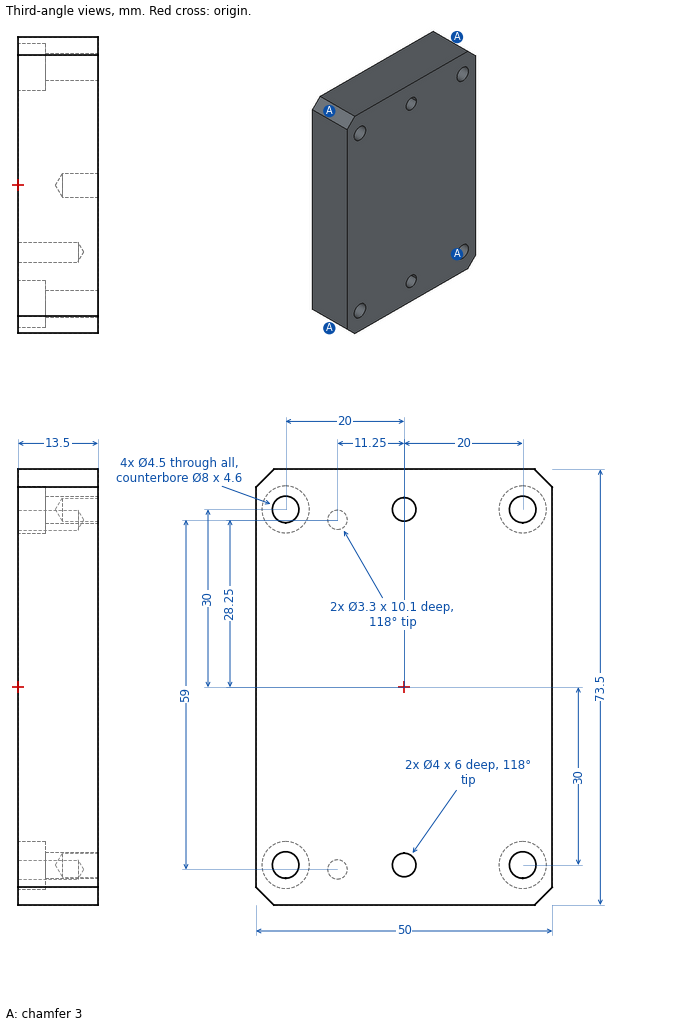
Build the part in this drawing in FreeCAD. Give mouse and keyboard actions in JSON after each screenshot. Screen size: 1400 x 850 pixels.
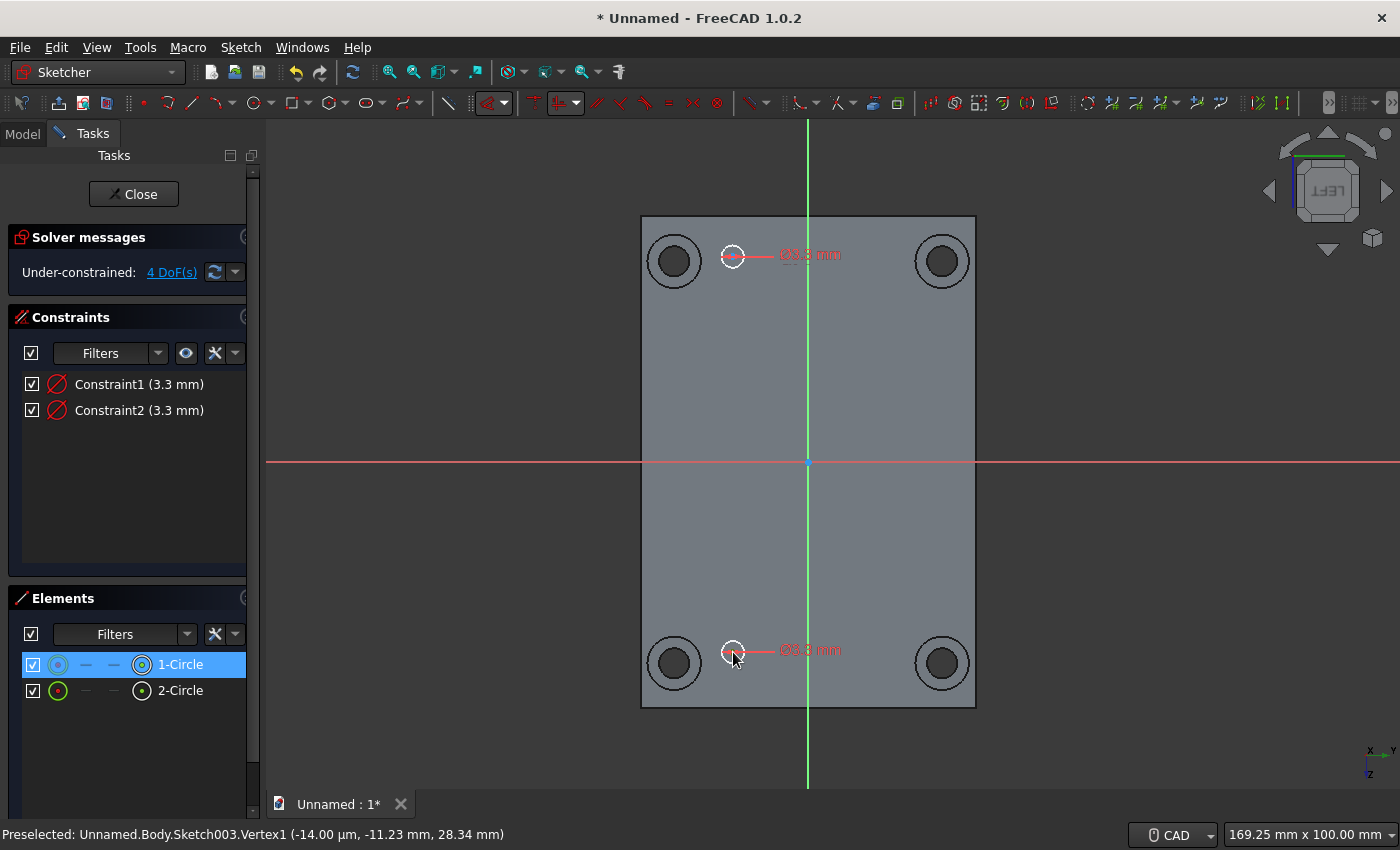
{"action": "left_click", "coordinate": [733, 257]}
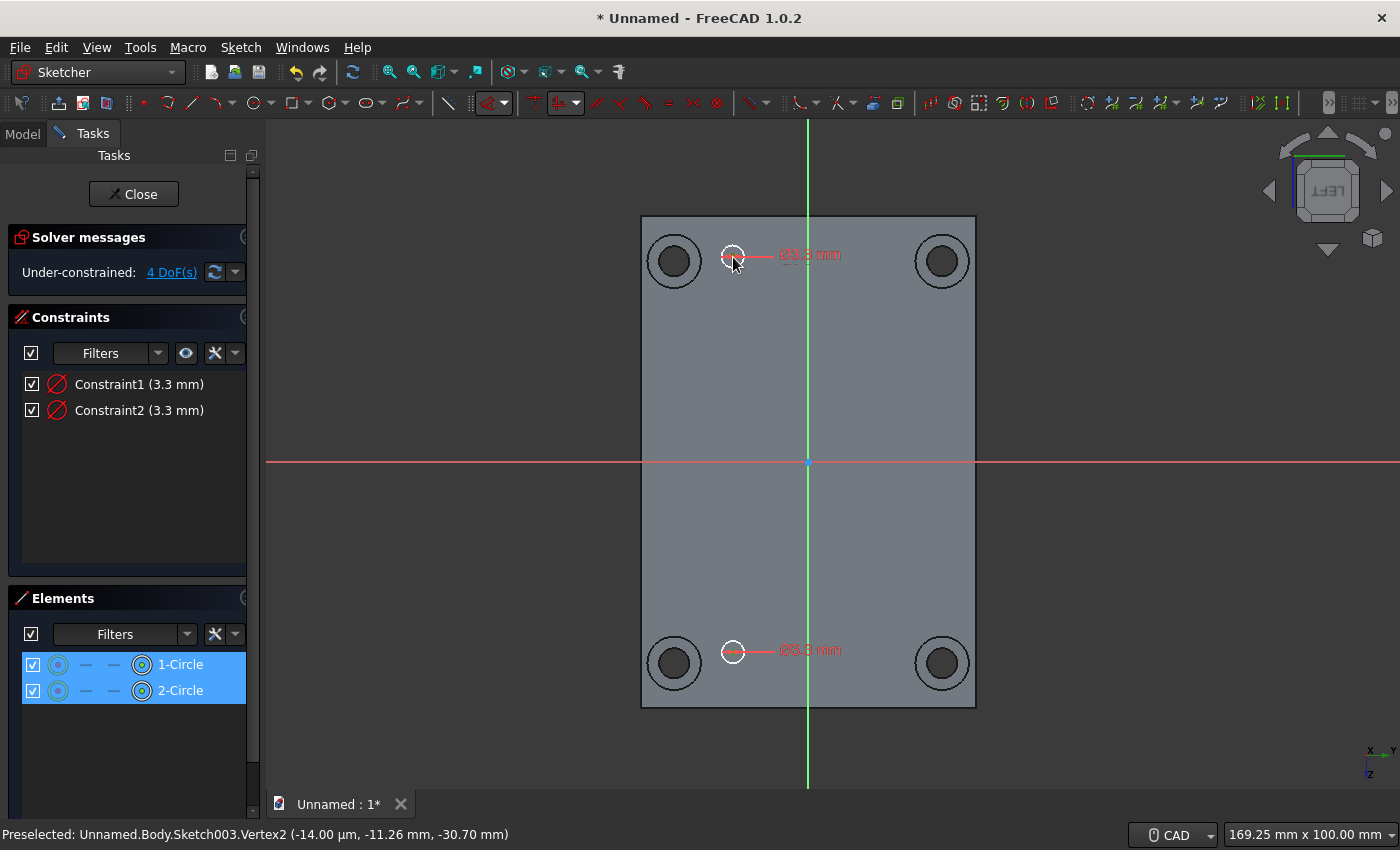
{"action": "key", "text": "v"}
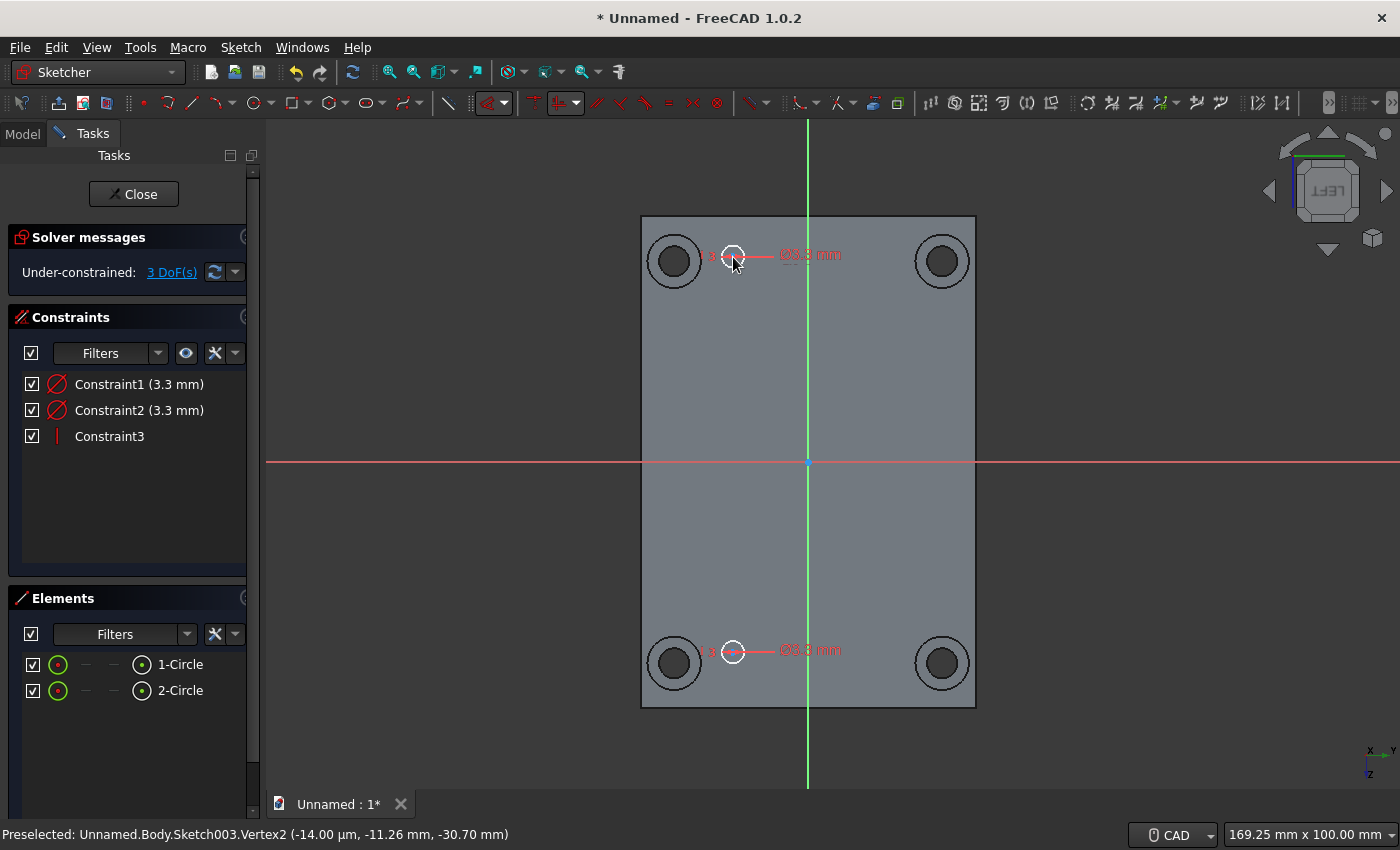
{"action": "left_click", "coordinate": [733, 652]}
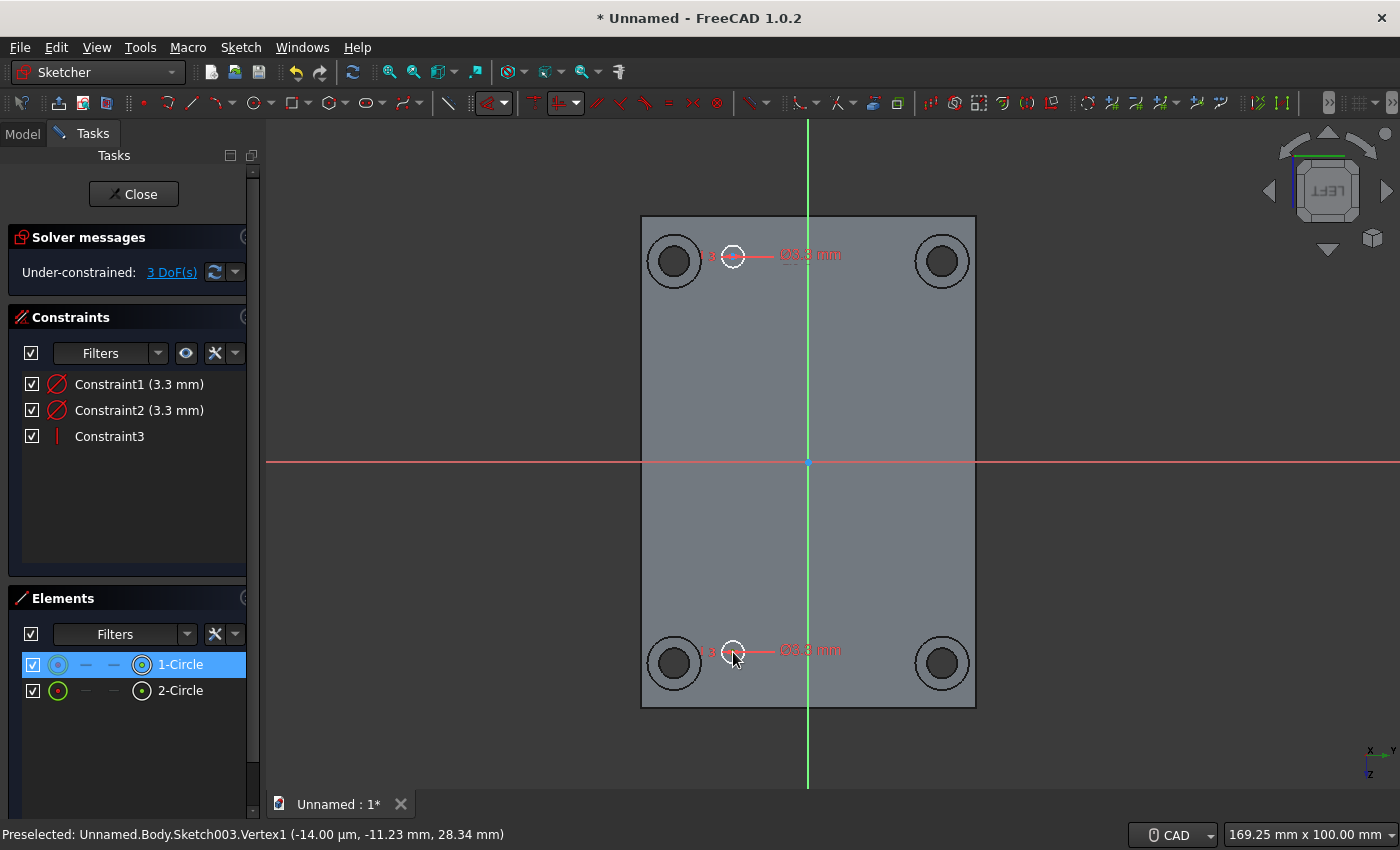
{"action": "left_click", "coordinate": [733, 257]}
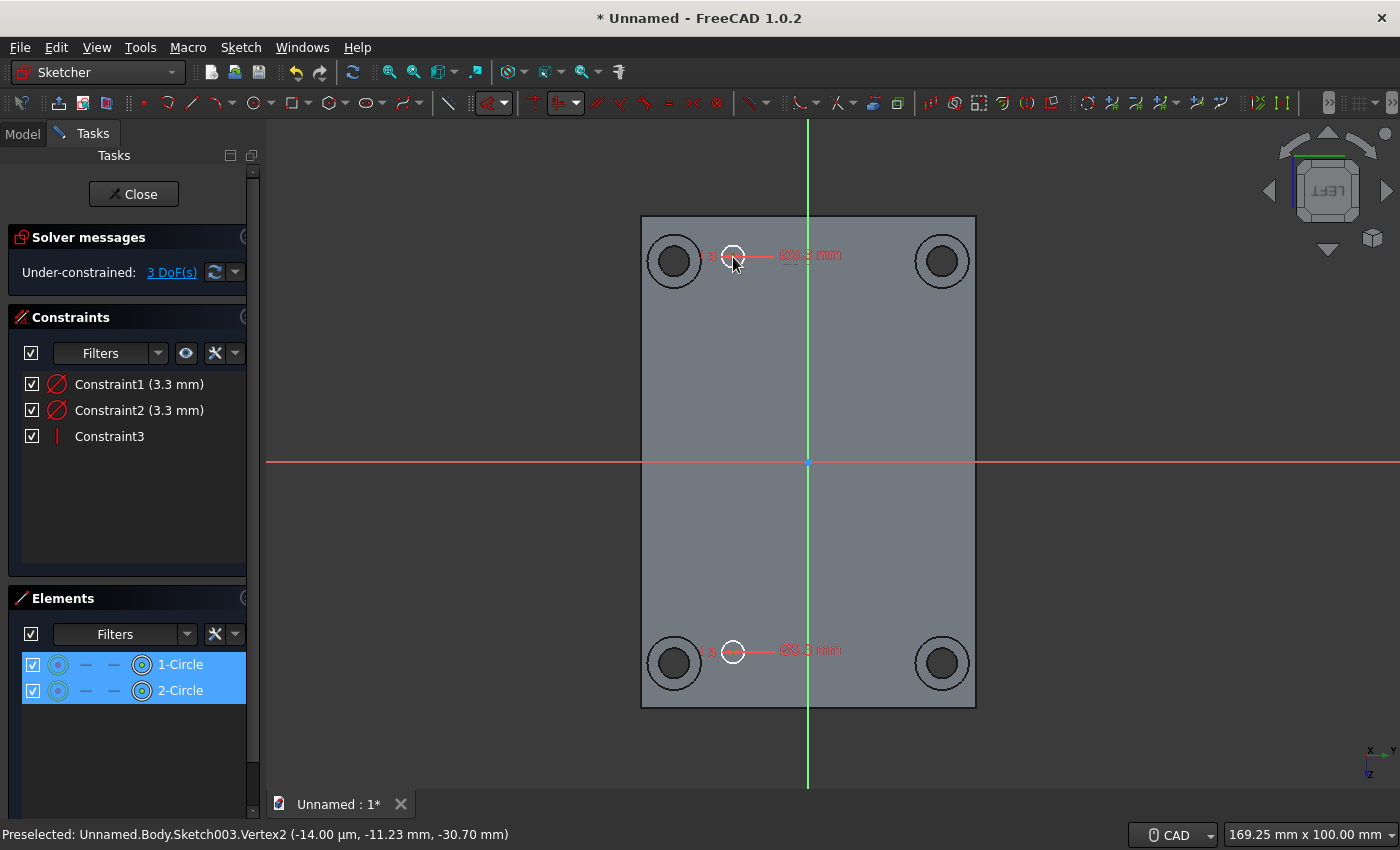
{"action": "left_click", "coordinate": [506, 104]}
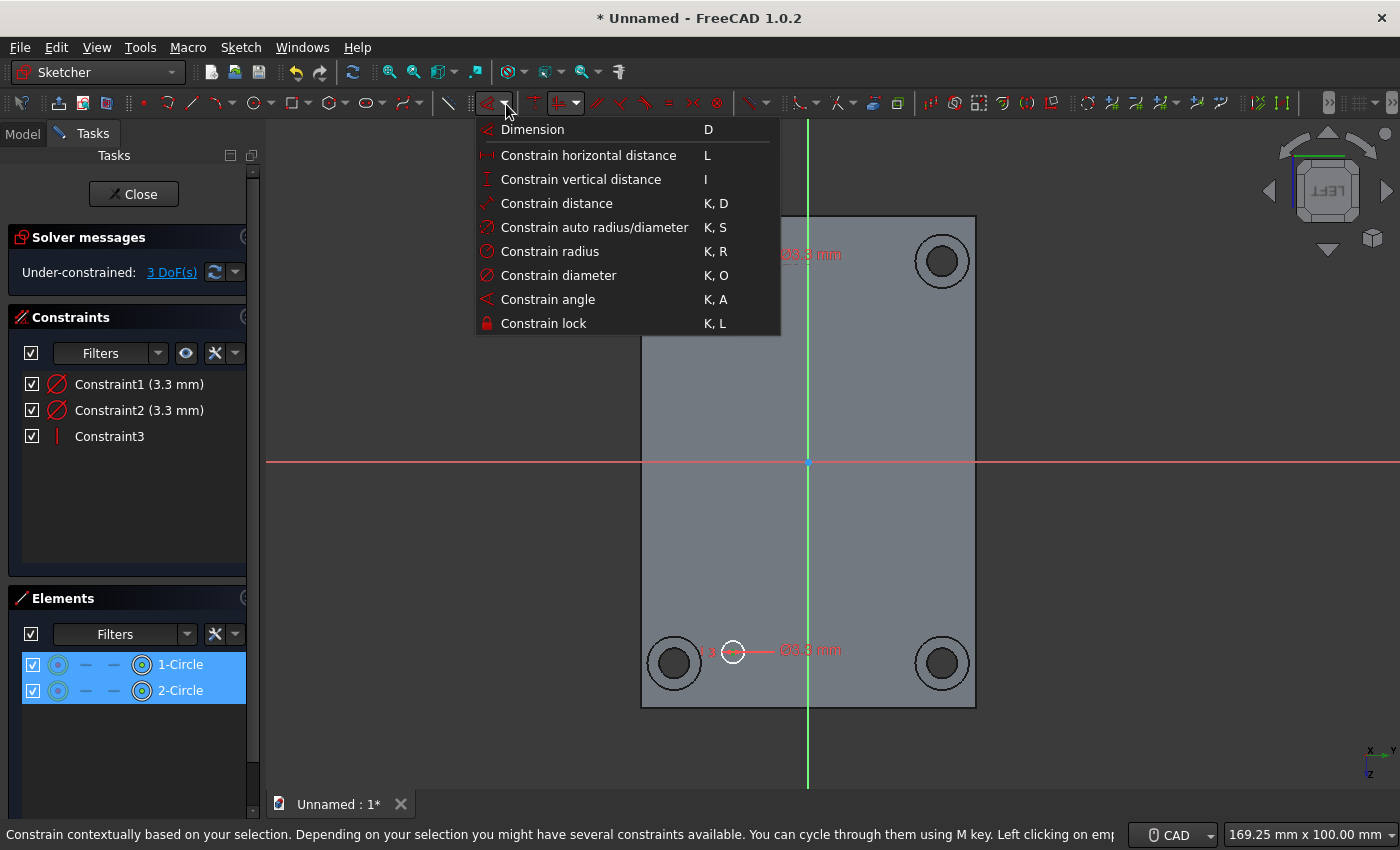
{"action": "left_click", "coordinate": [628, 179]}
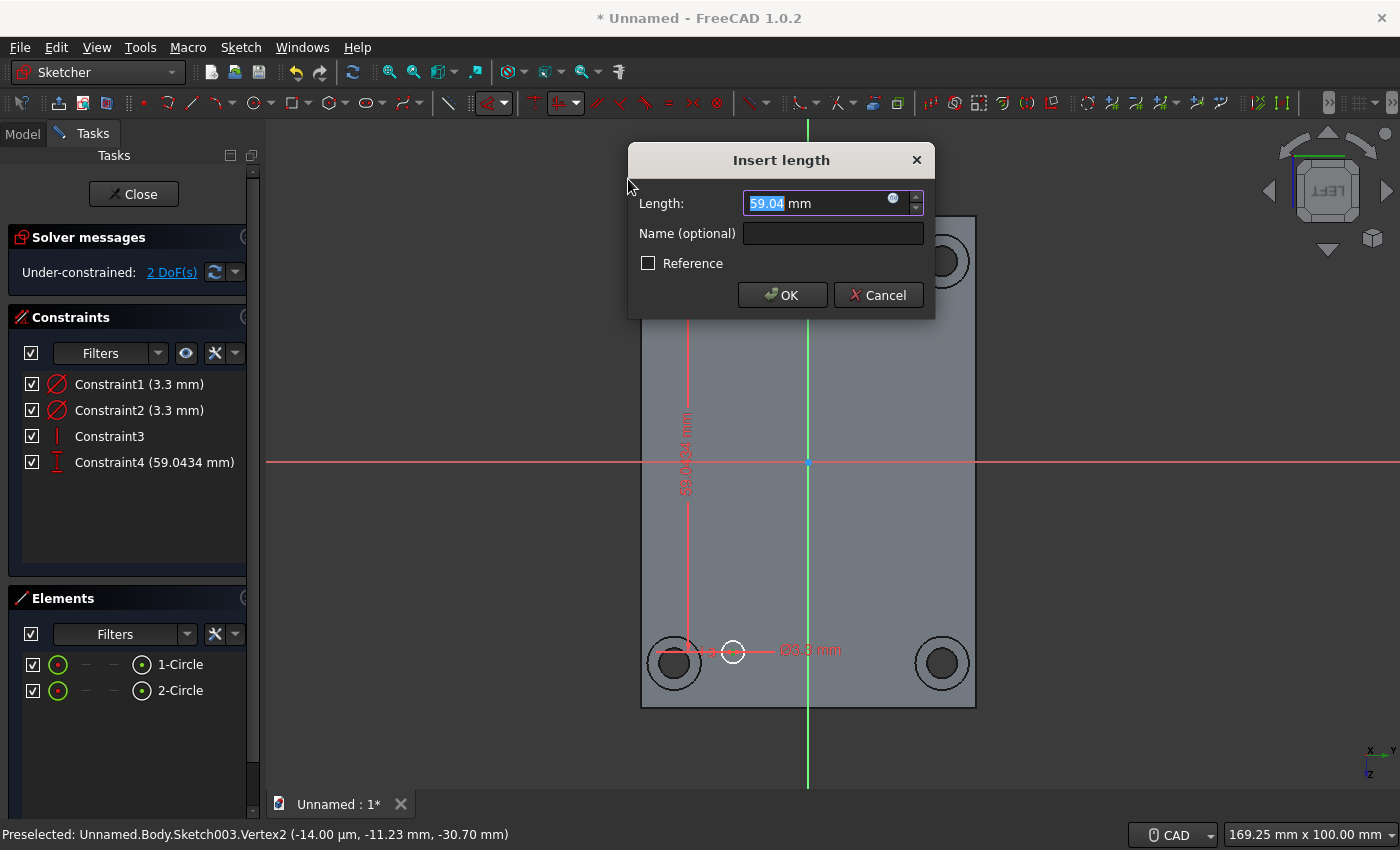
{"action": "type", "text": "59"}
{"action": "key", "text": "Return"}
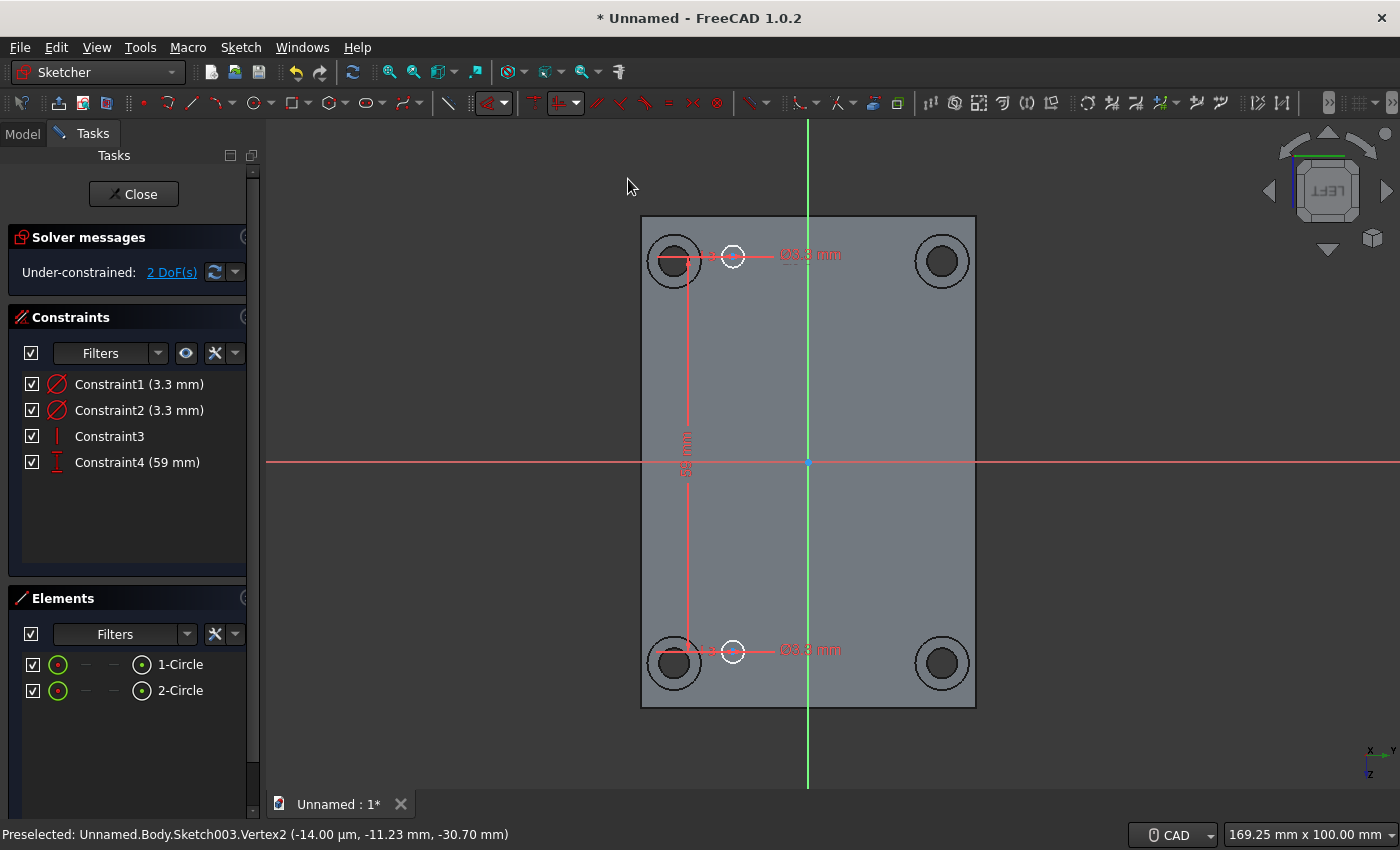
{"action": "left_click", "coordinate": [733, 652]}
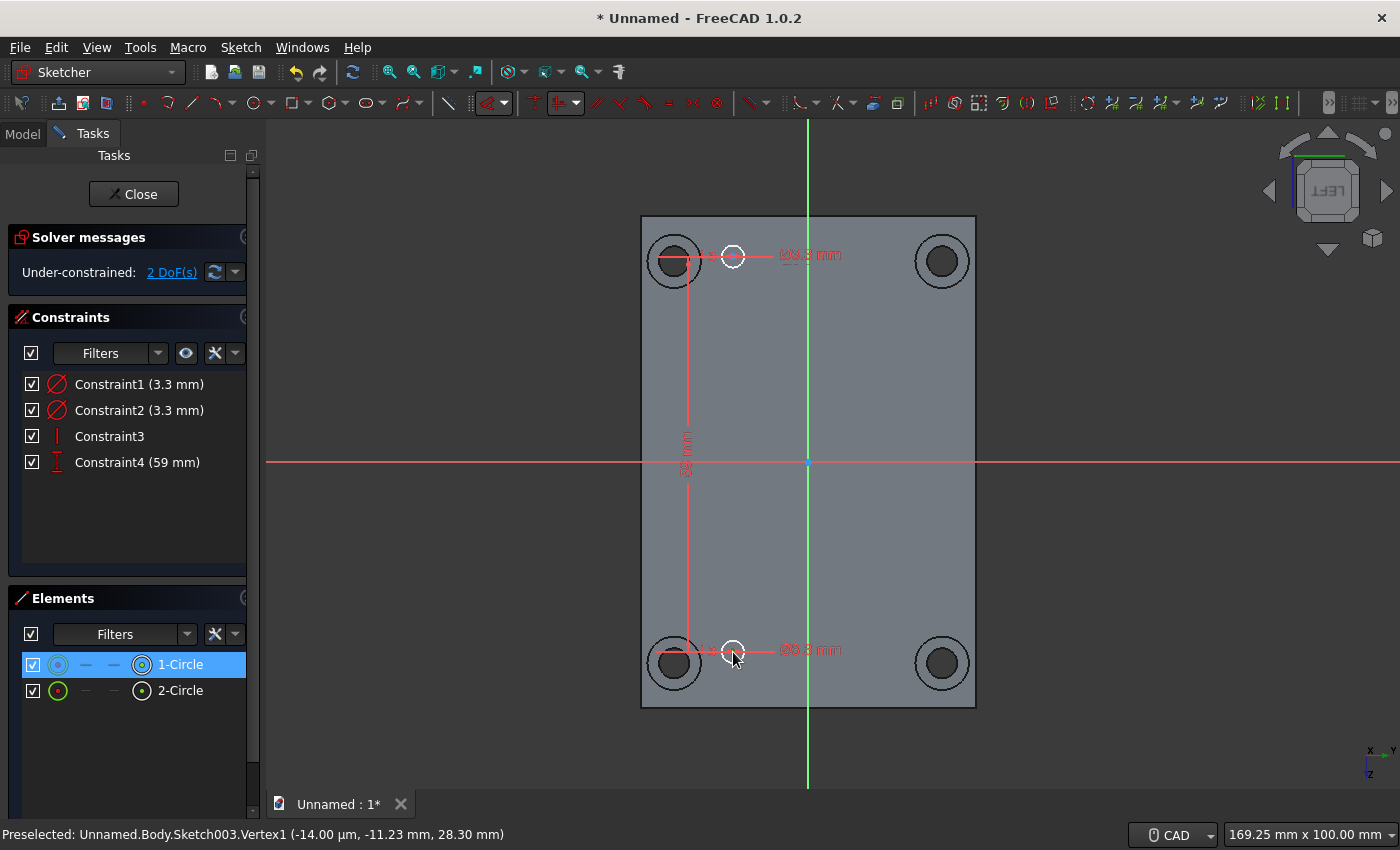
{"action": "key", "text": "l"}